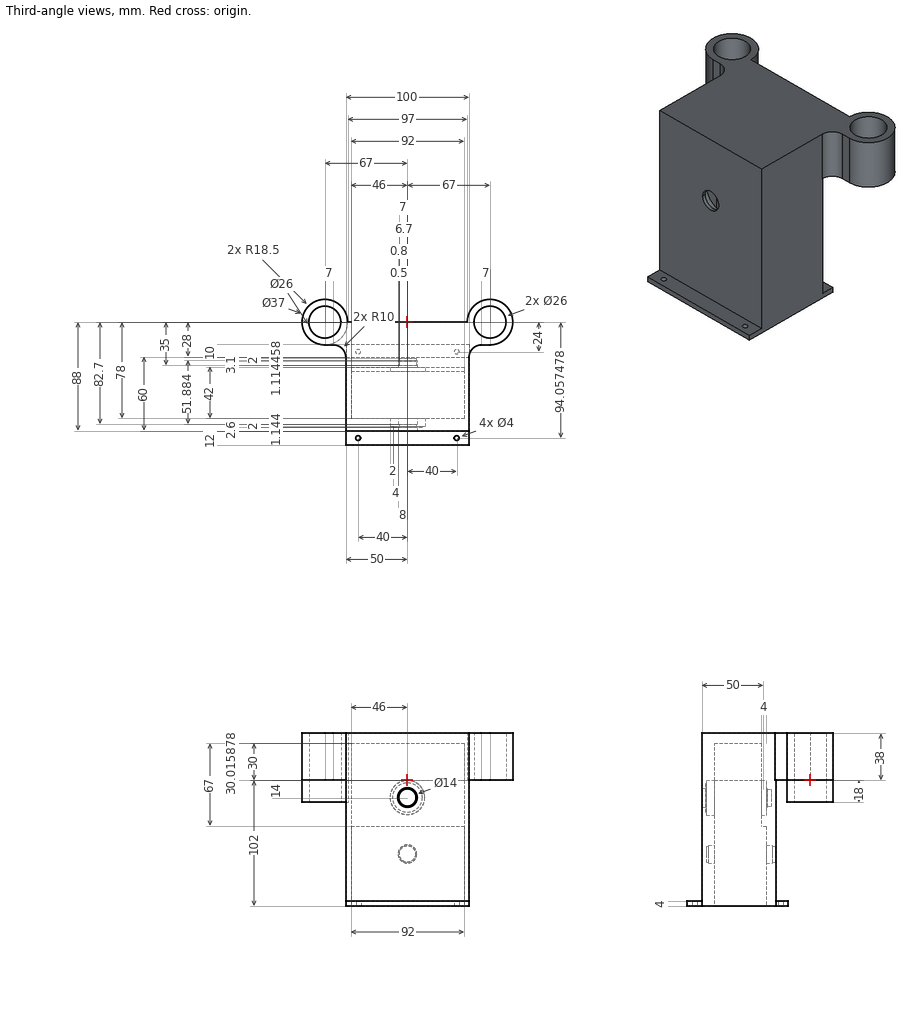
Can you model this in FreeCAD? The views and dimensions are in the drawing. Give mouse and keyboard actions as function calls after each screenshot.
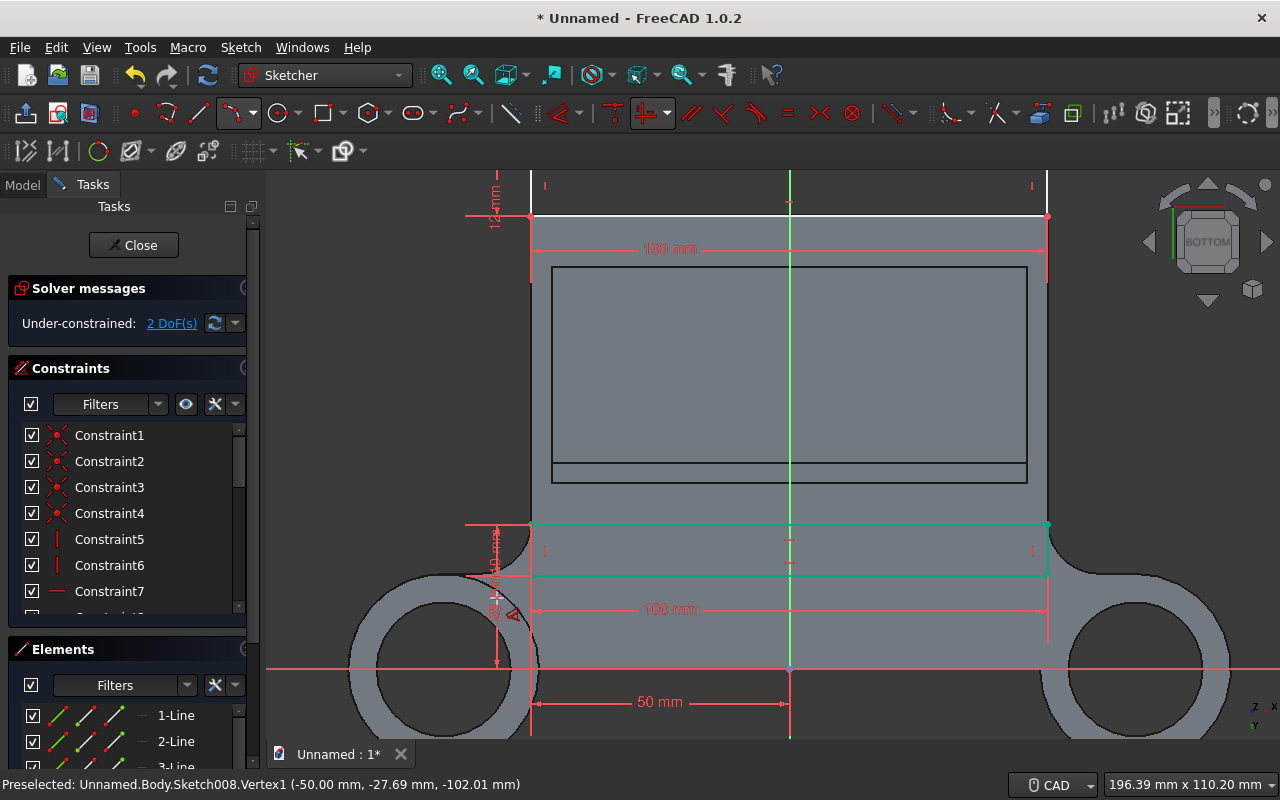
scroll(531, 543, down, 2)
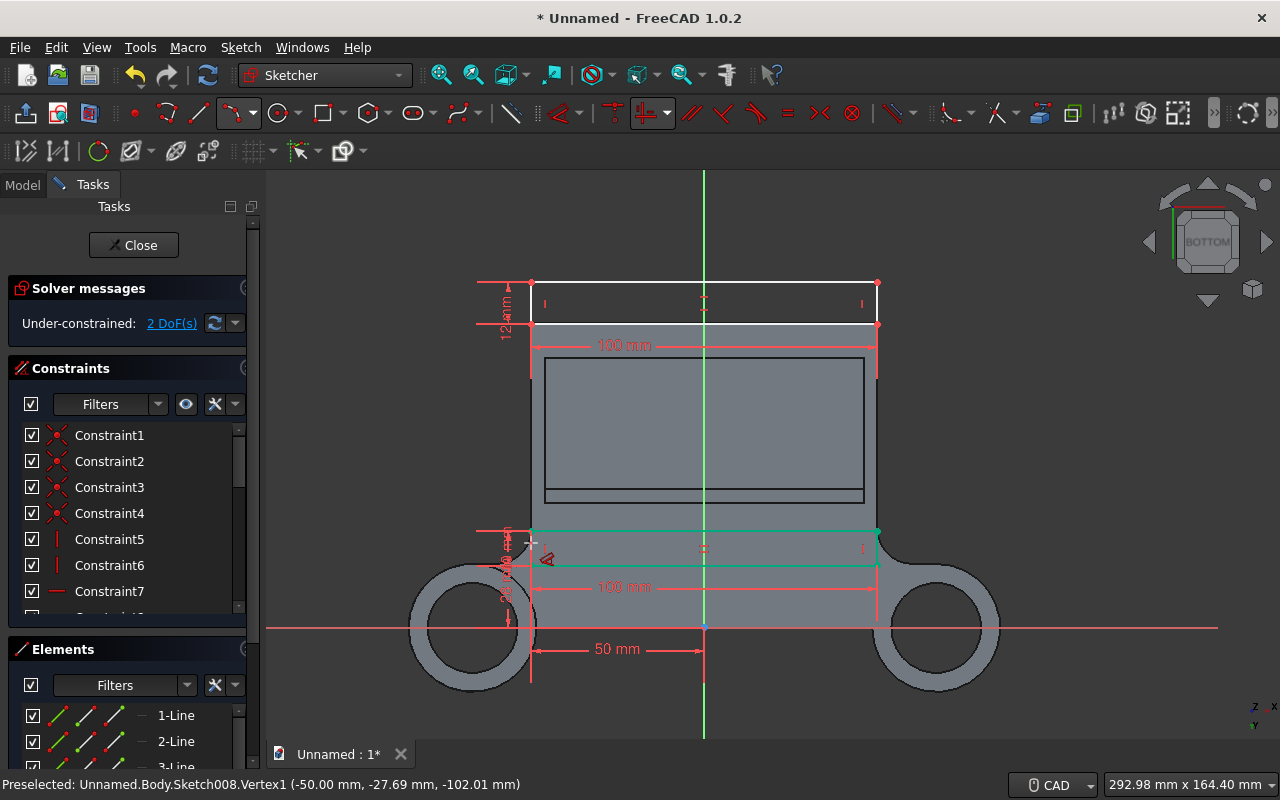
click(531, 282)
click(618, 248)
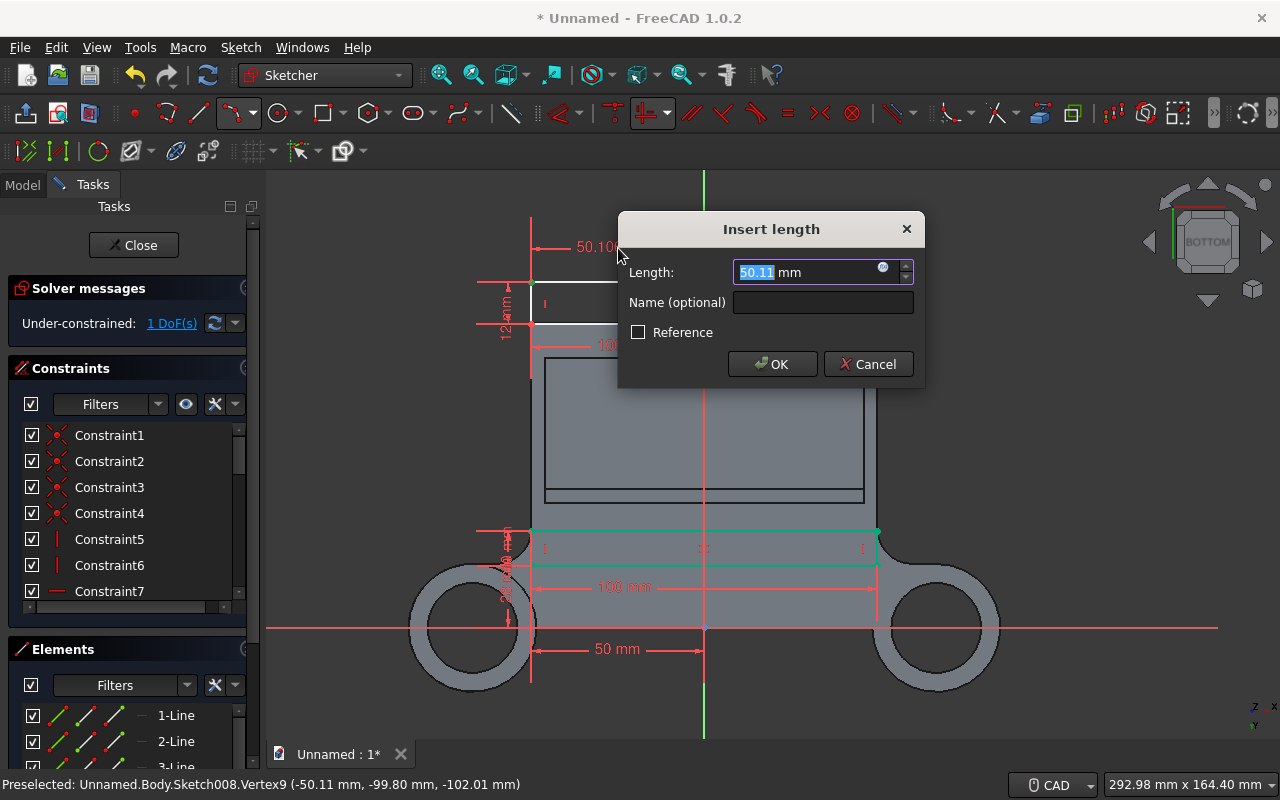
text(50)
key(Return)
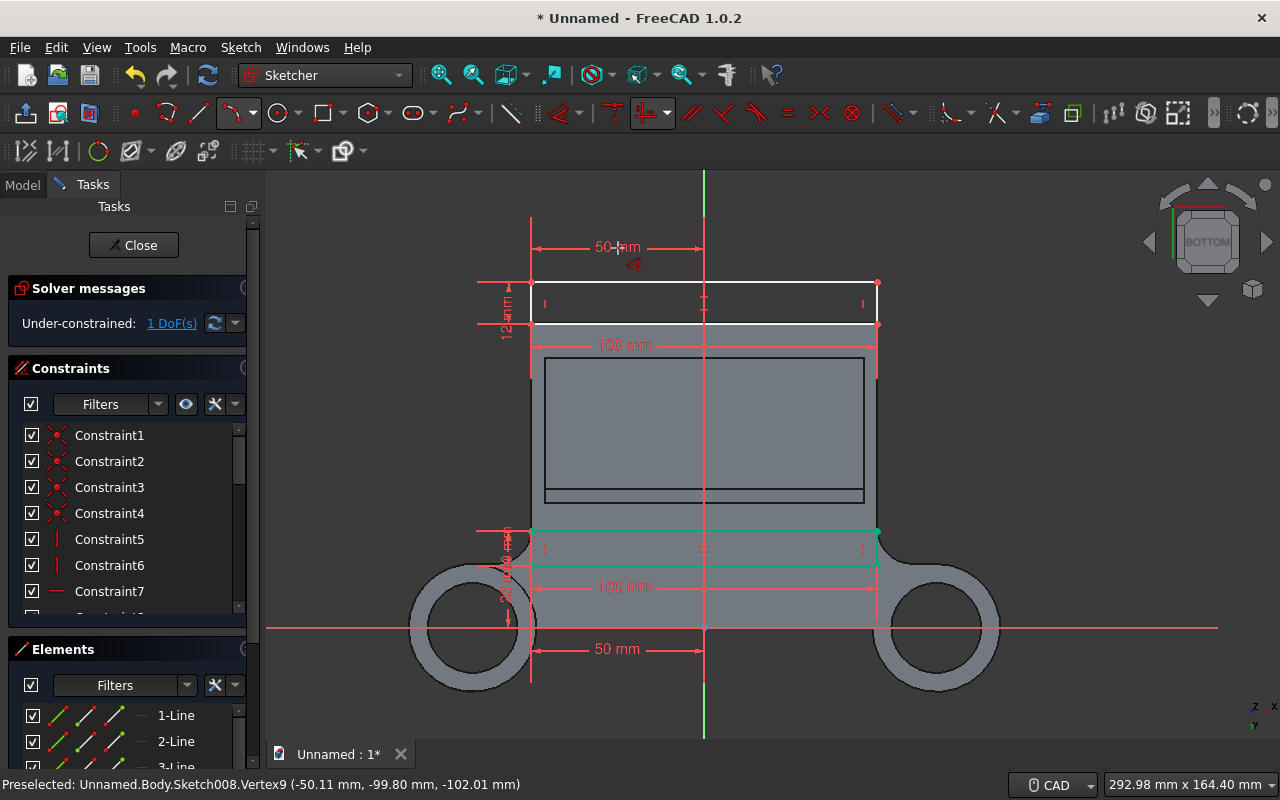
click(531, 324)
click(497, 476)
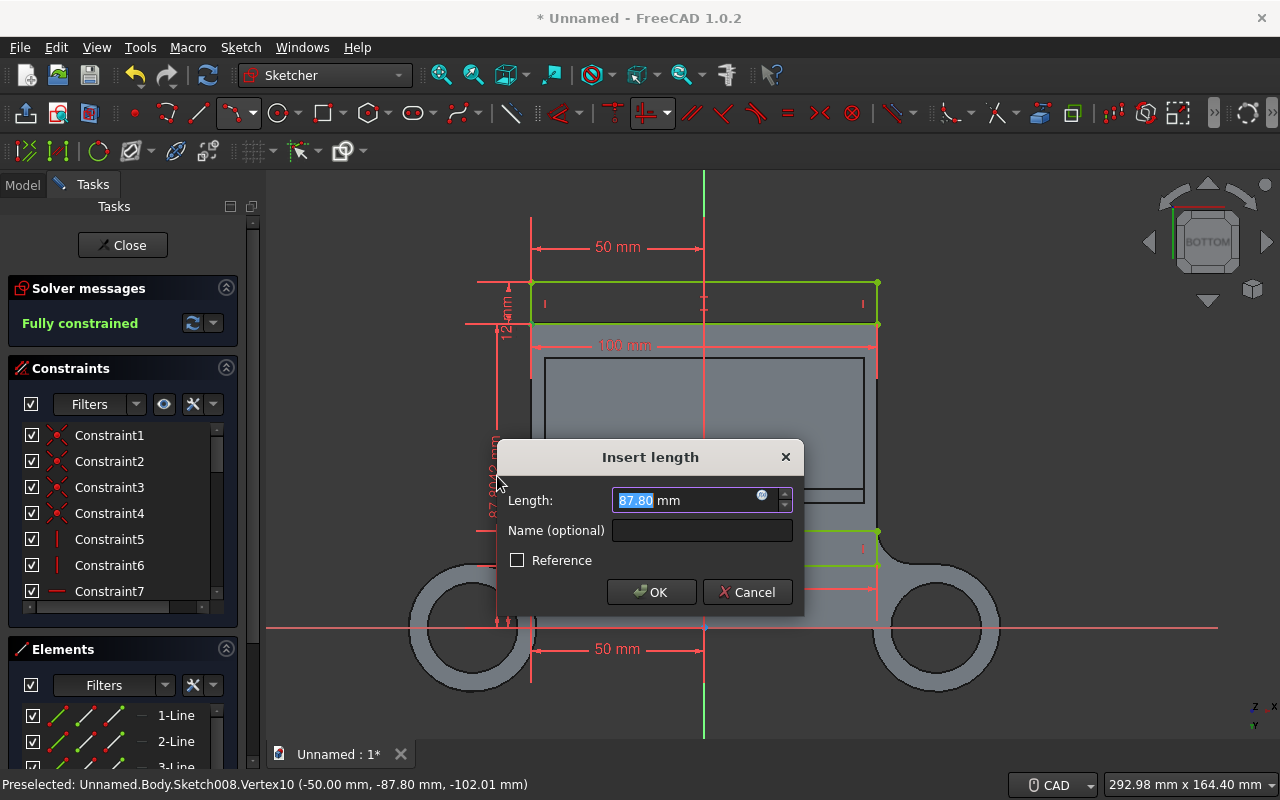
text(88)
key(Return)
key(Escape)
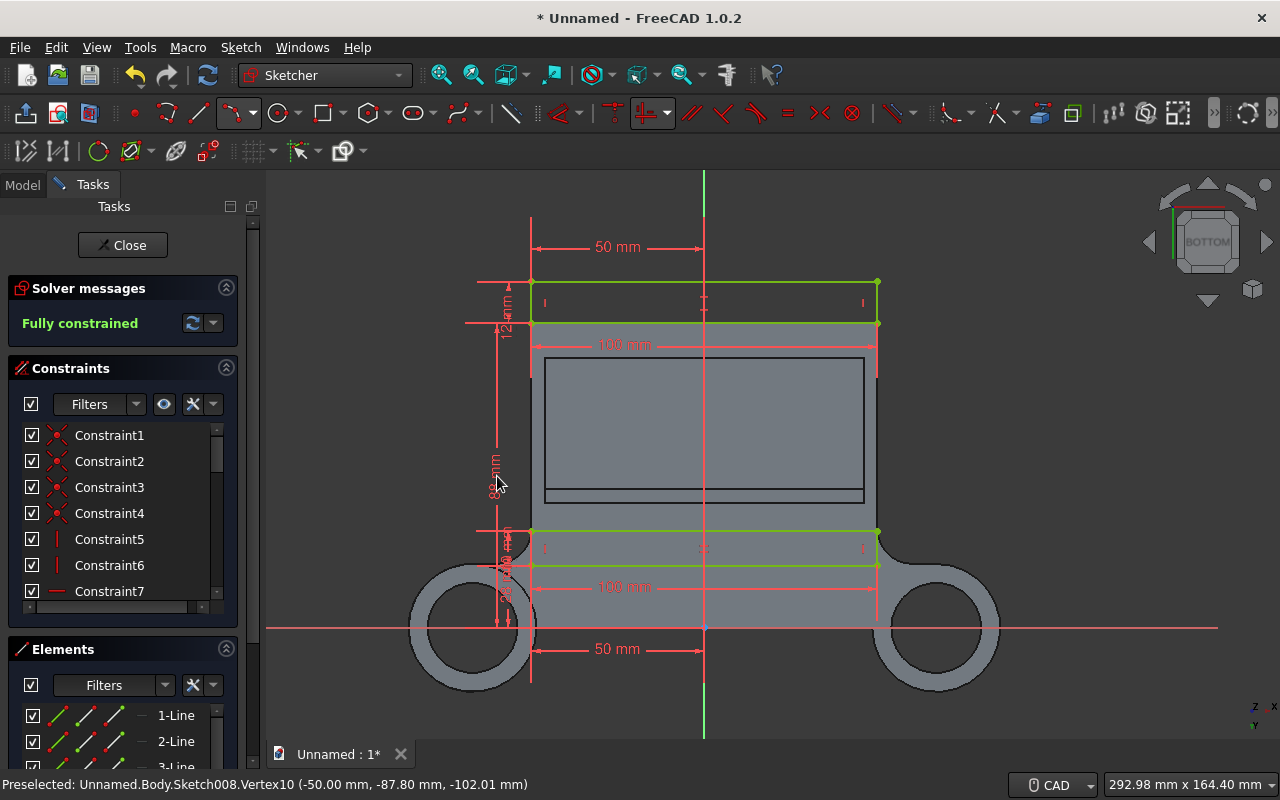
click(123, 245)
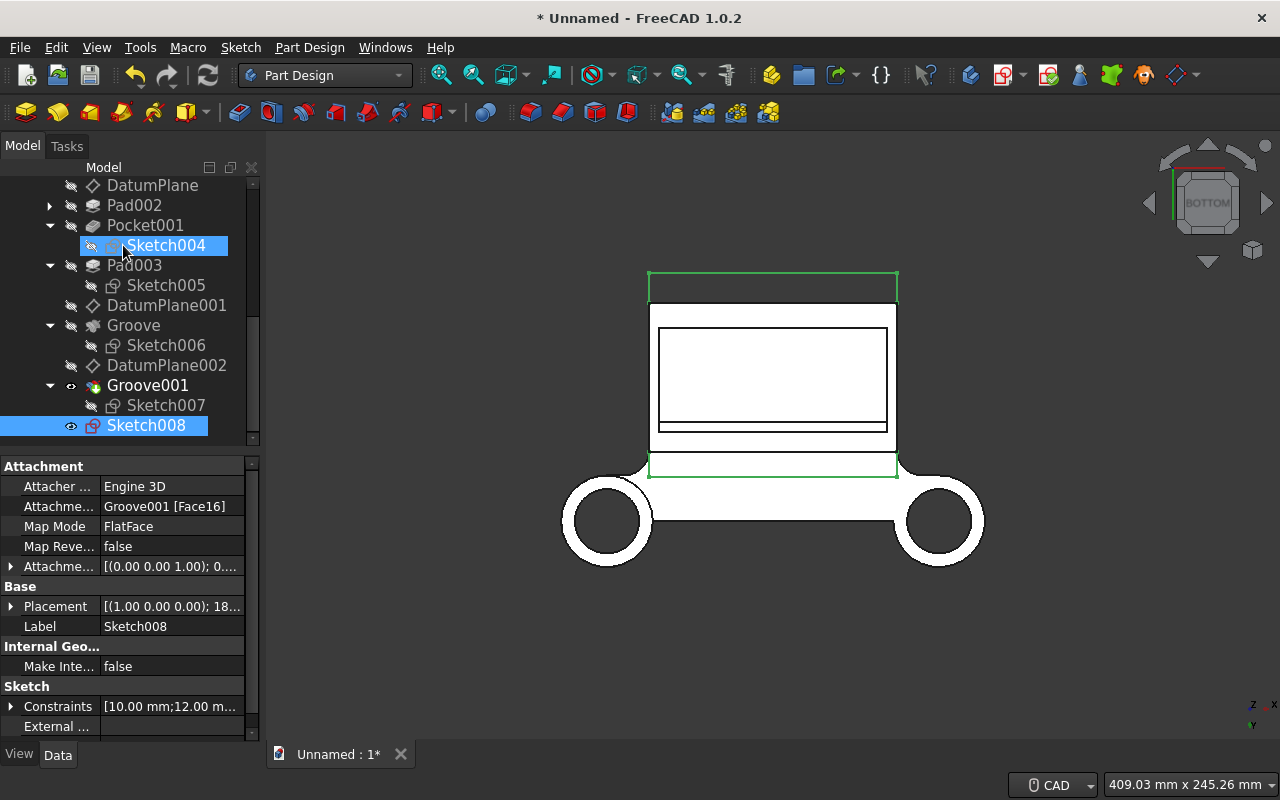
click(26, 112)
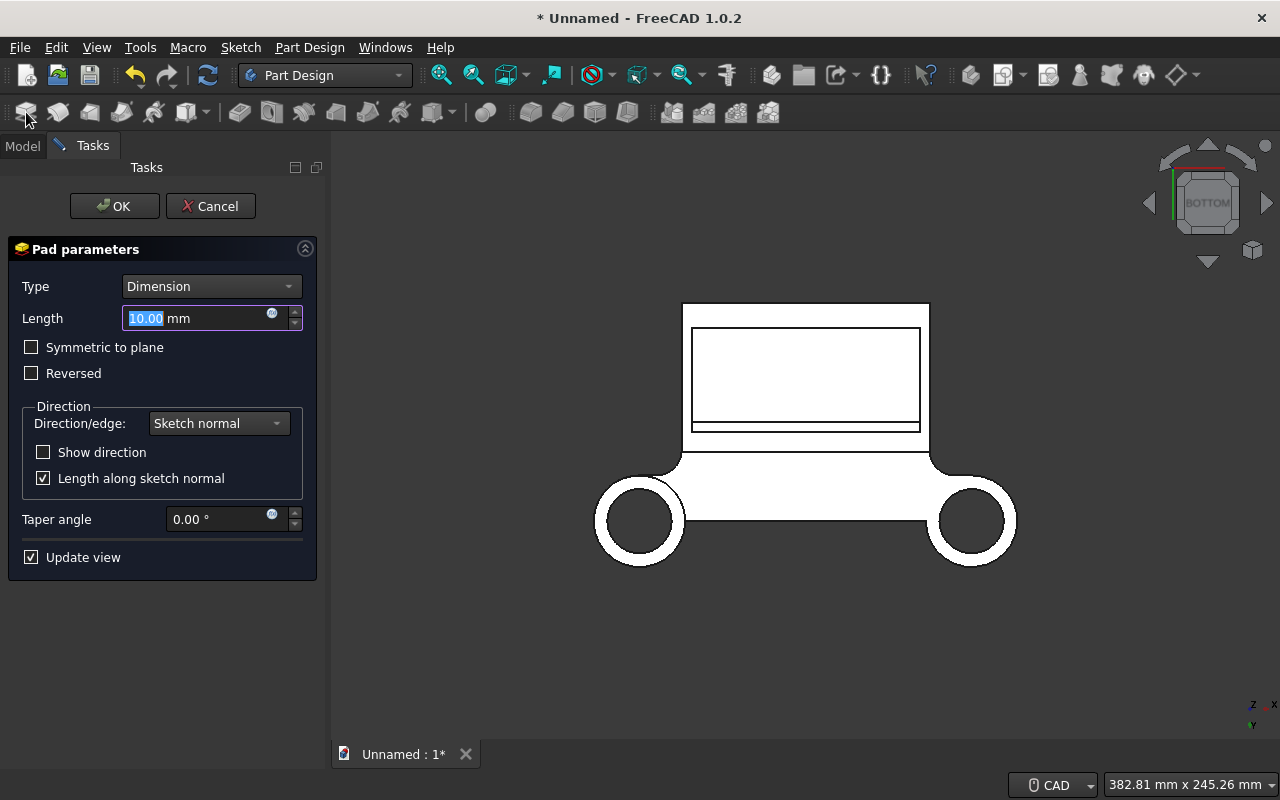
text(4)
key(Tab)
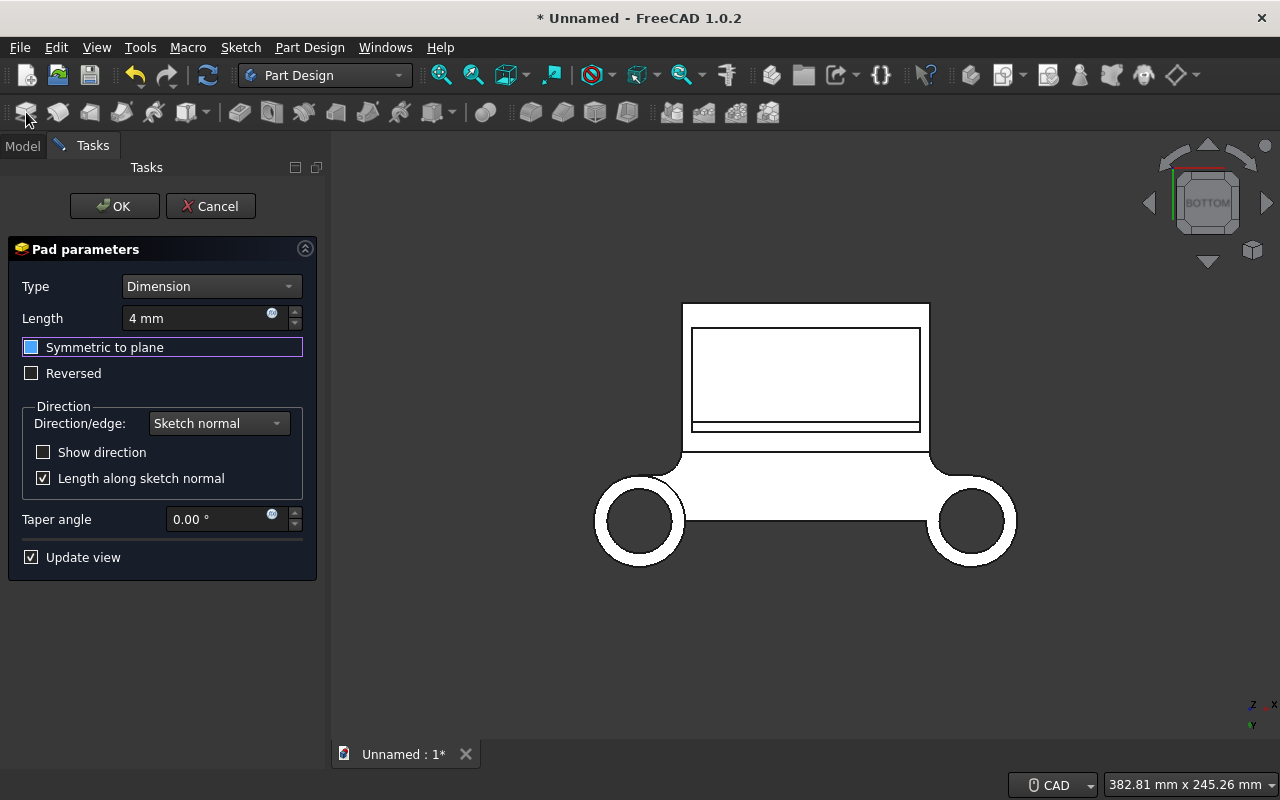
click(30, 373)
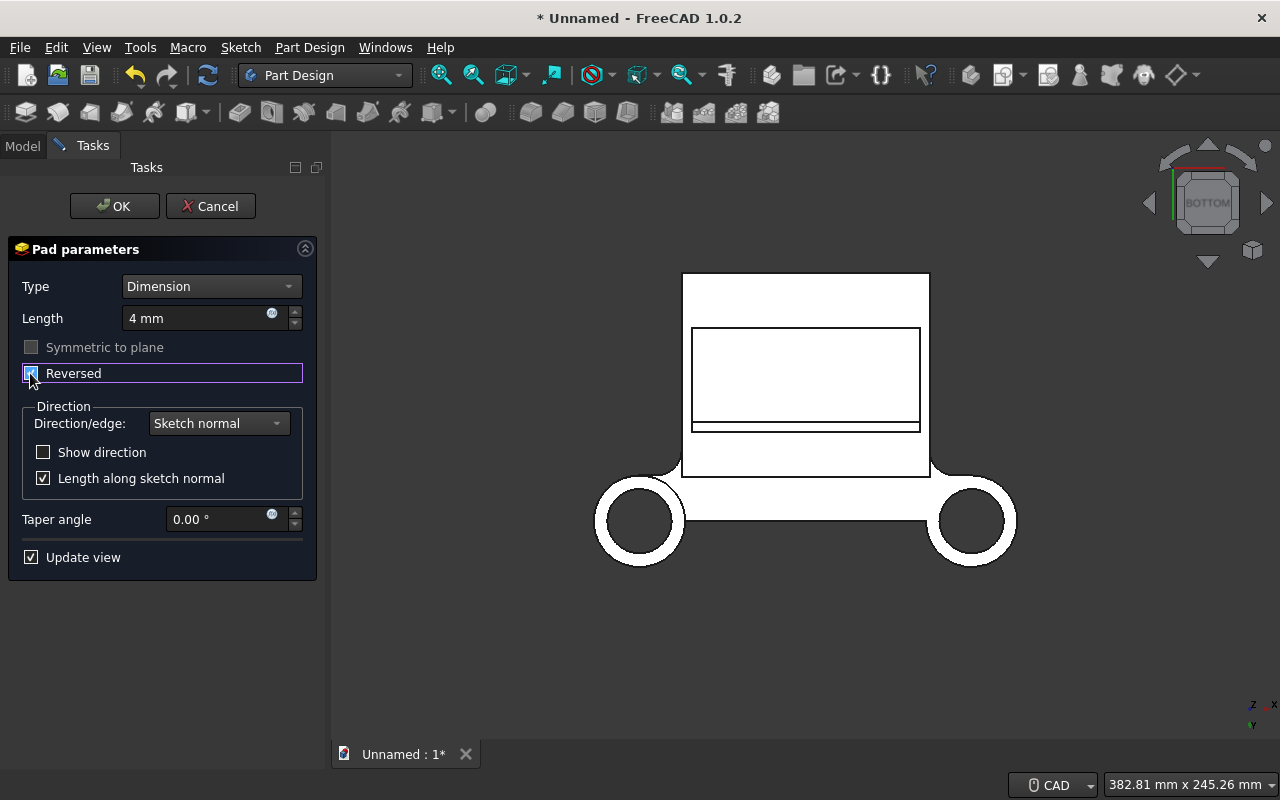
click(115, 206)